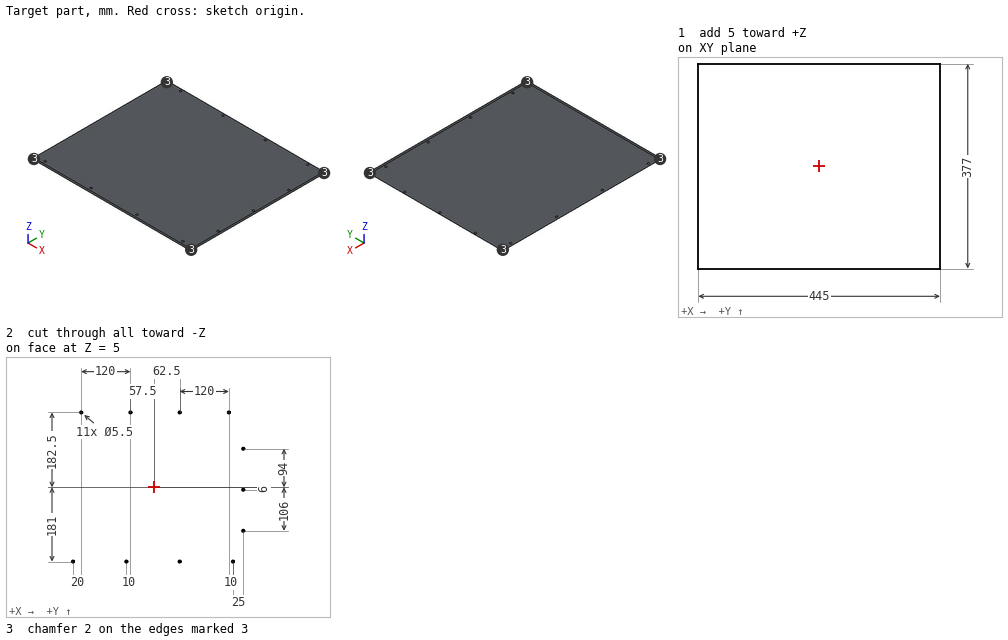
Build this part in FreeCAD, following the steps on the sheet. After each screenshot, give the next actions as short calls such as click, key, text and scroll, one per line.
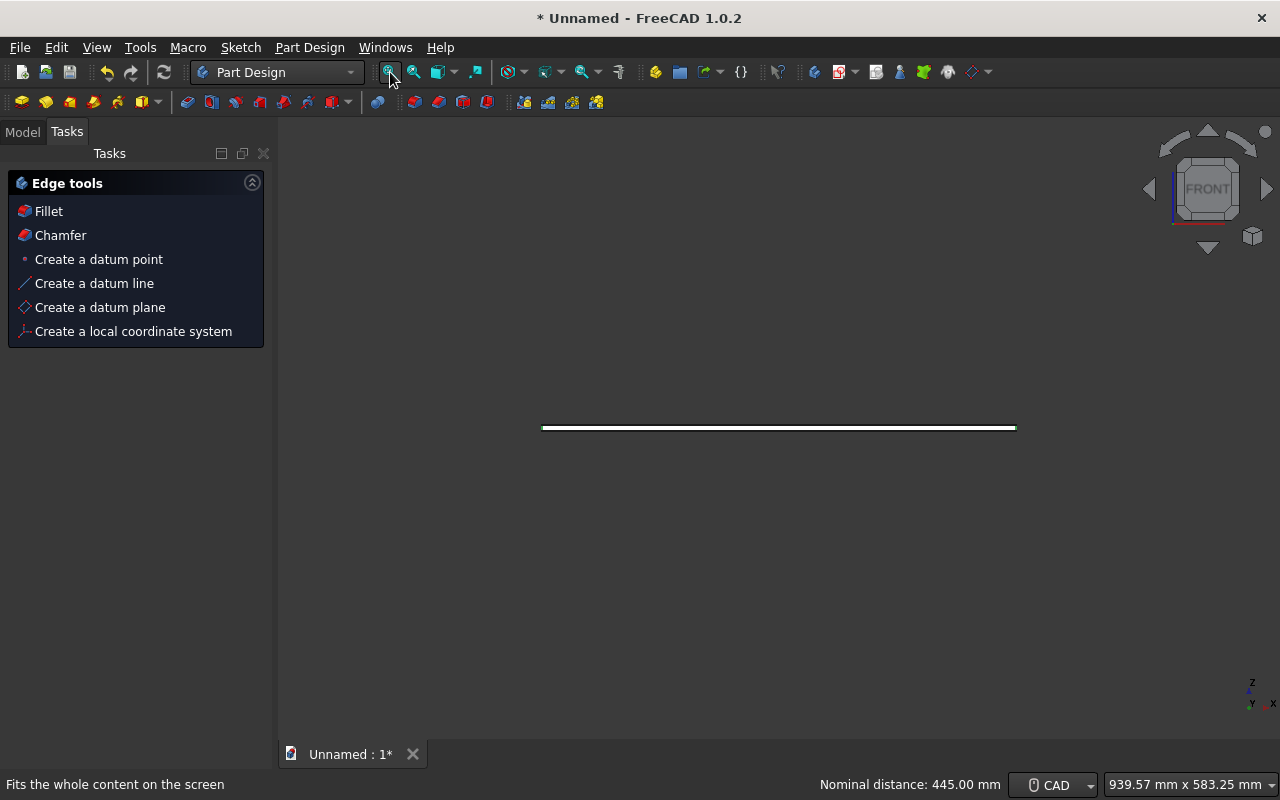
key(3)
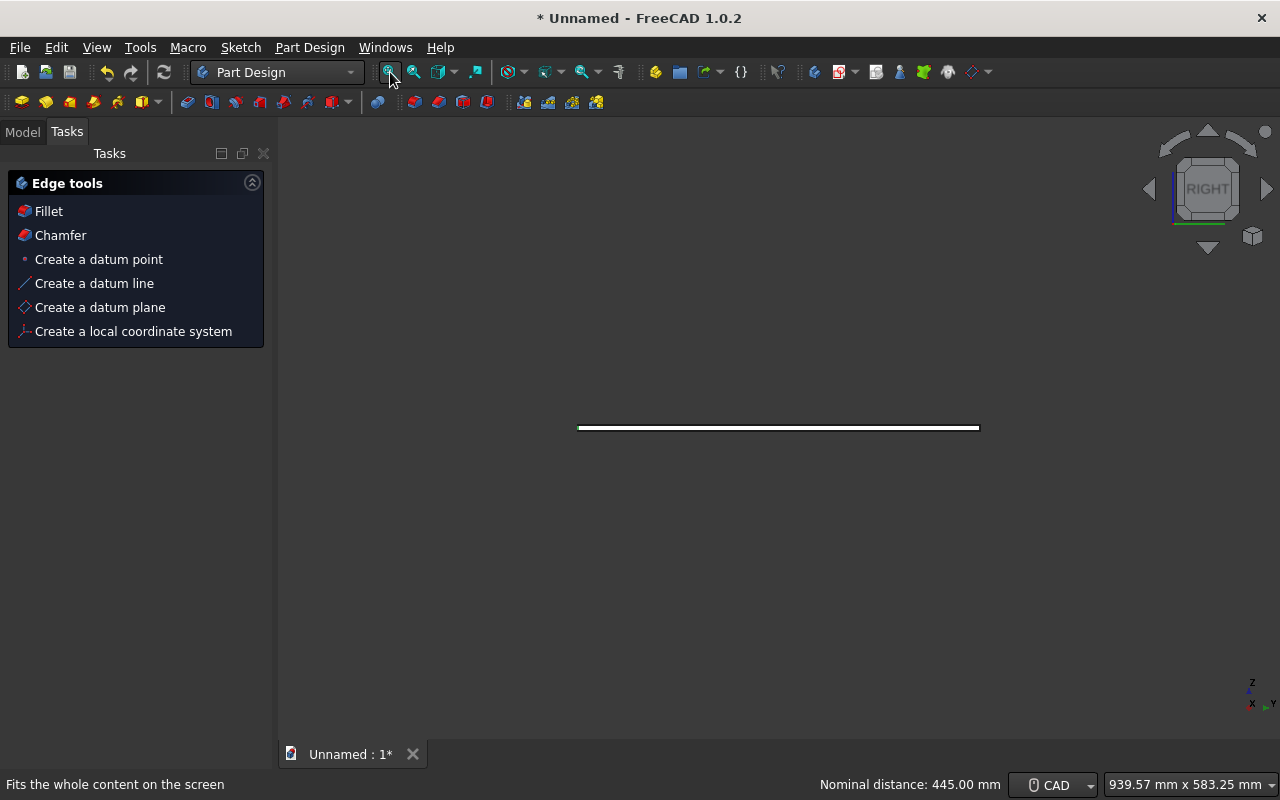
click(390, 72)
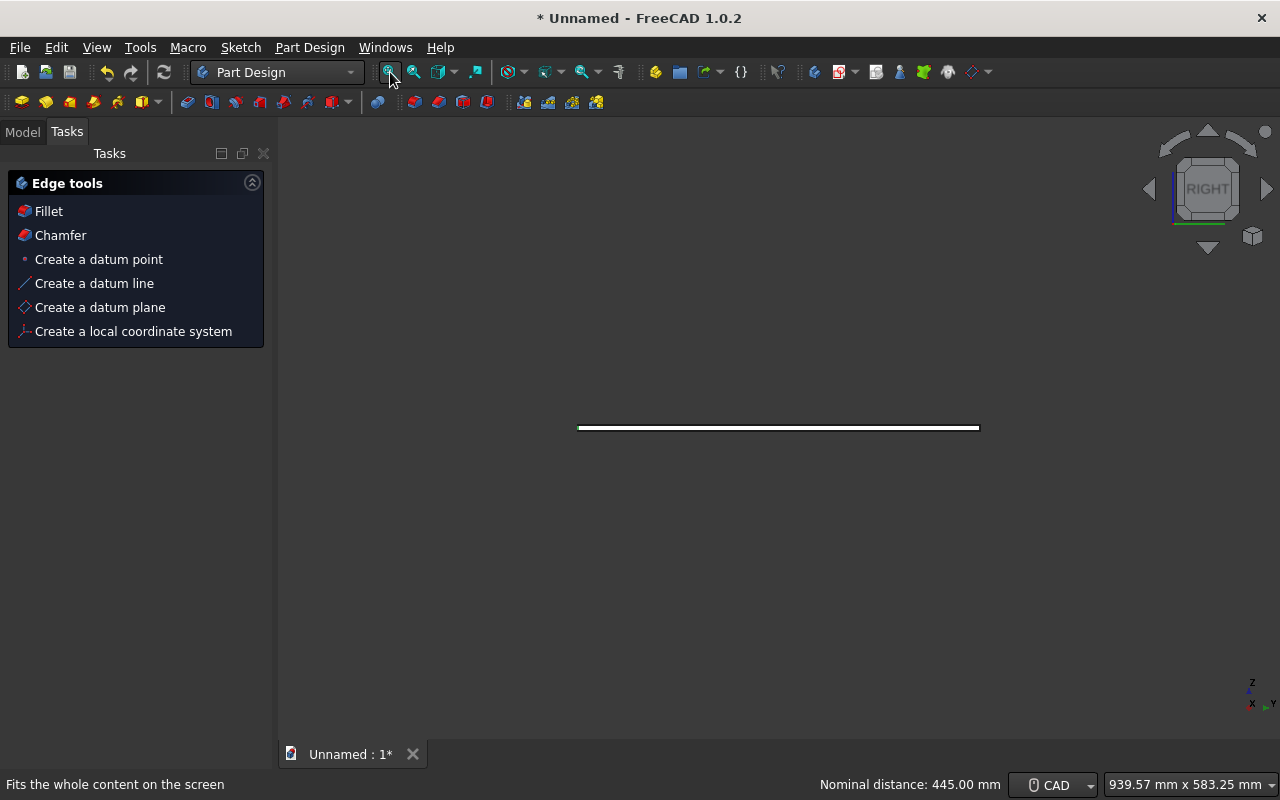
scroll(980, 427, up, 11)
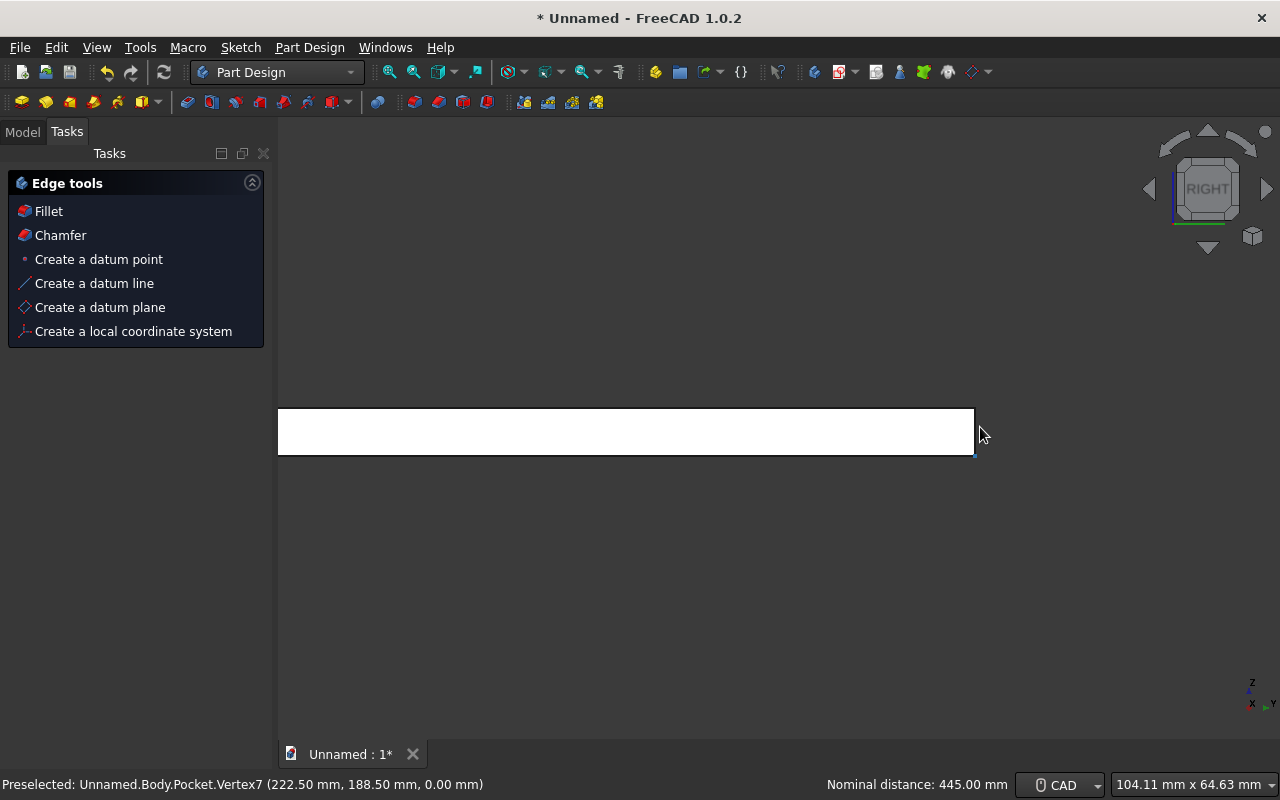
click(975, 431, ctrl)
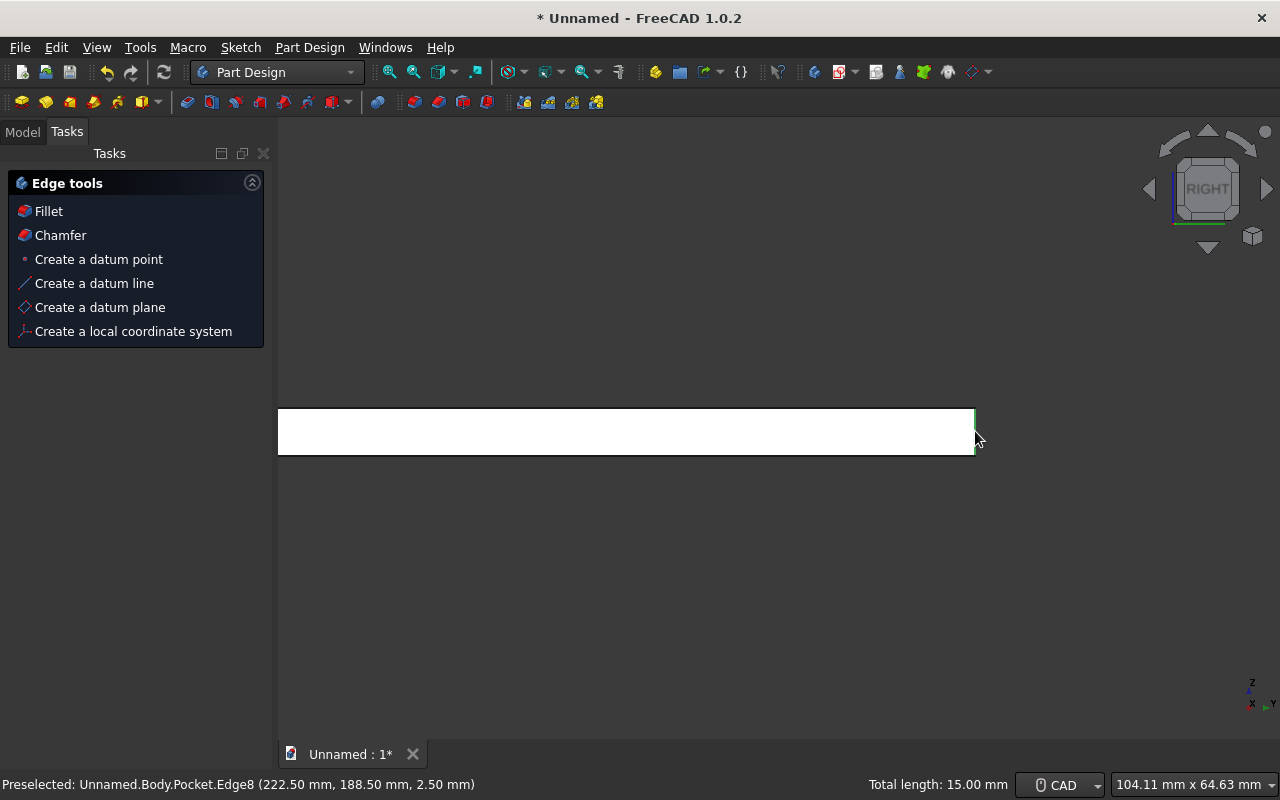
click(390, 72)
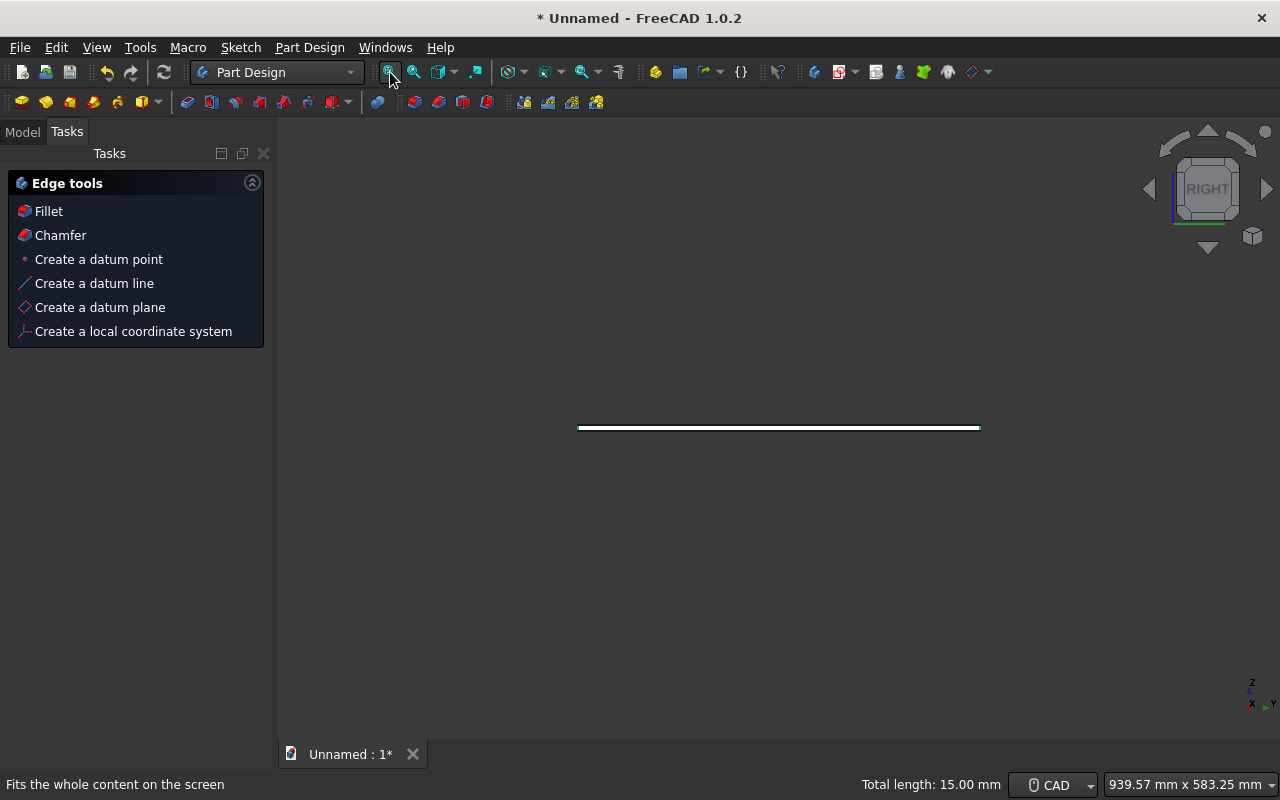
key(5)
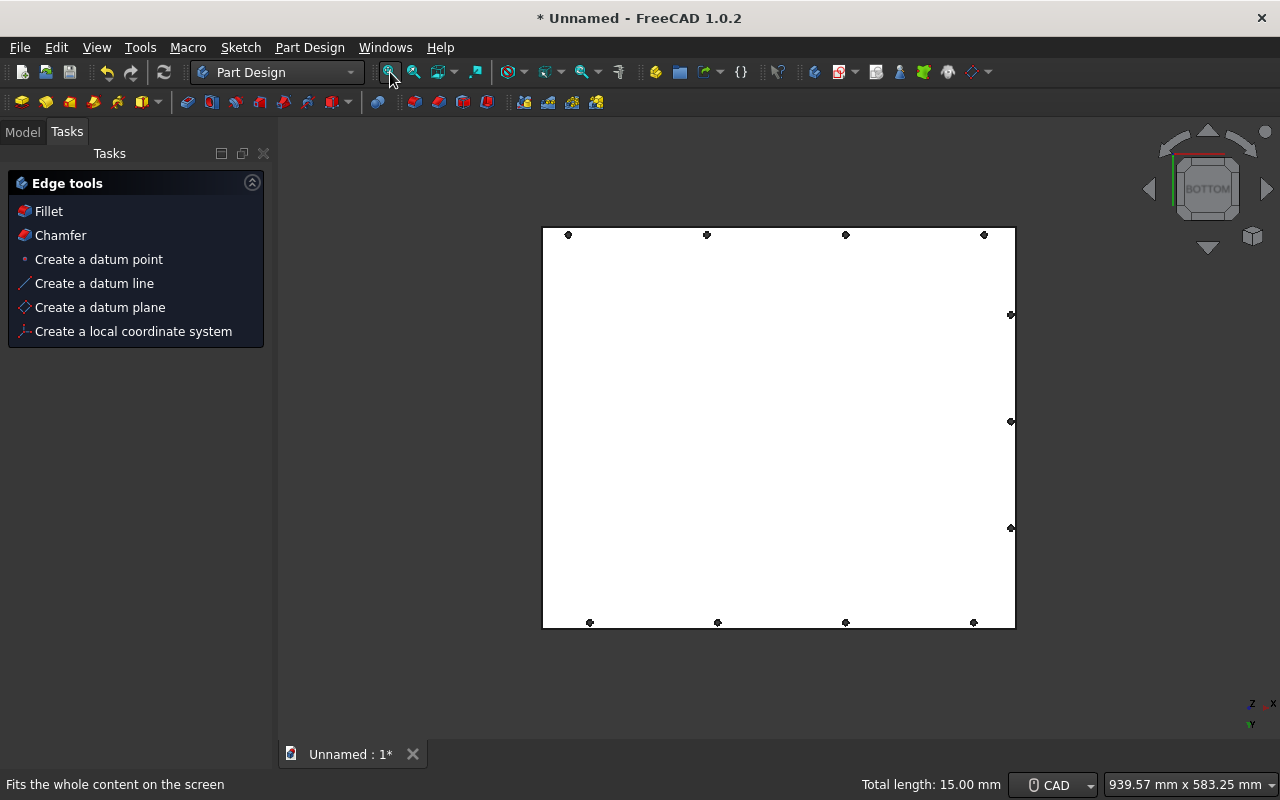
scroll(542, 628, up, 11)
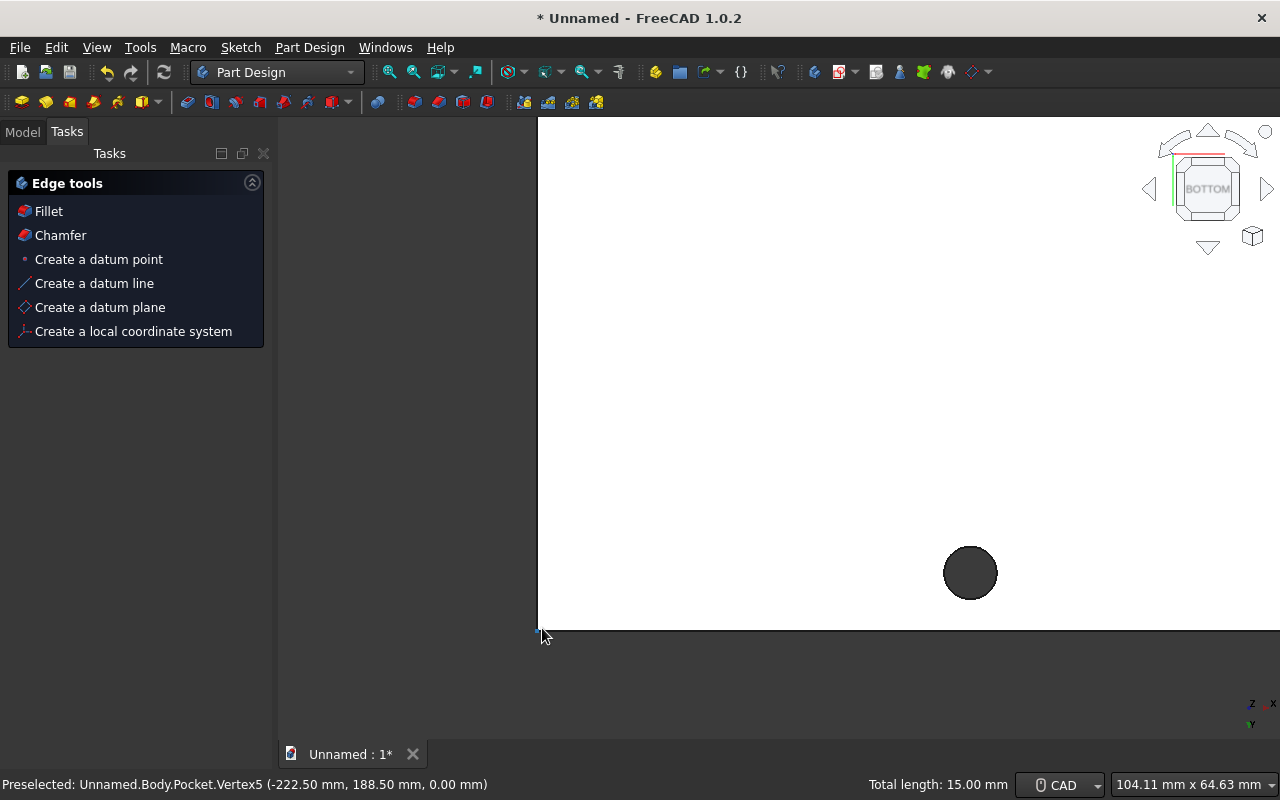
key(v)
key(f)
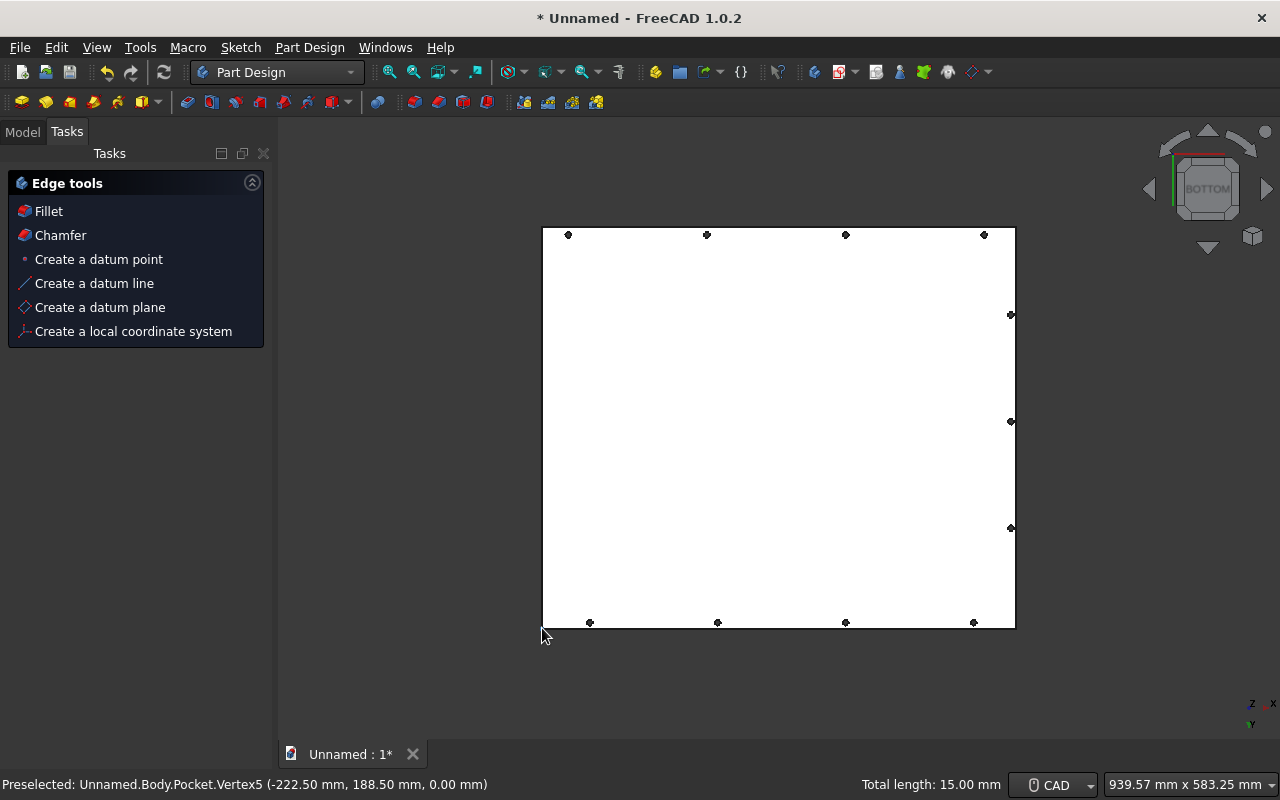
key(4)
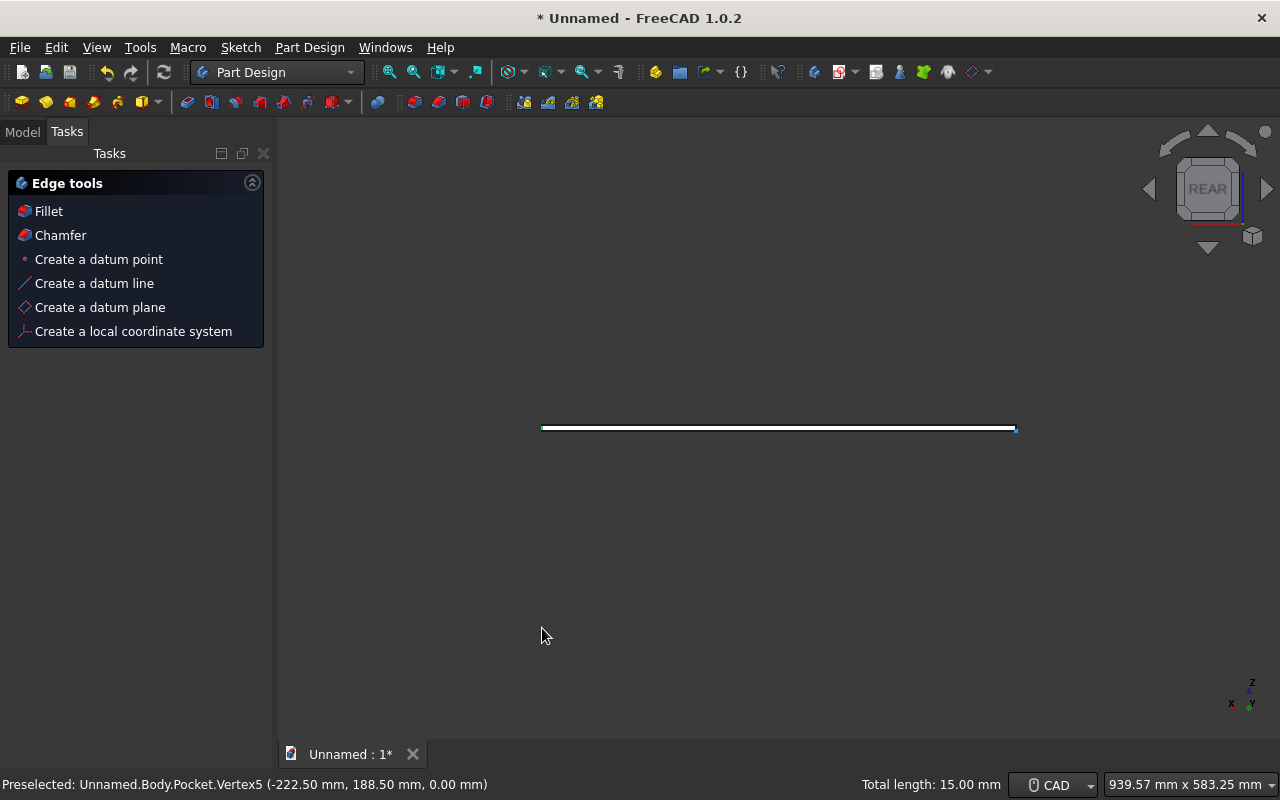
scroll(1016, 427, up, 11)